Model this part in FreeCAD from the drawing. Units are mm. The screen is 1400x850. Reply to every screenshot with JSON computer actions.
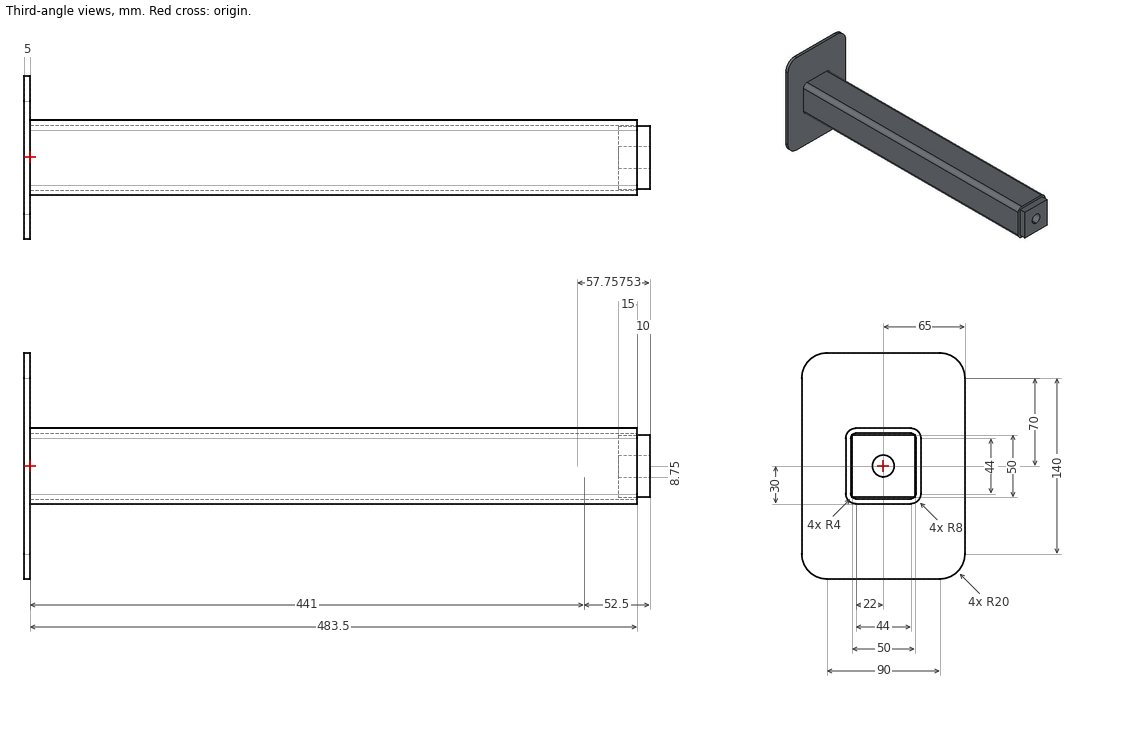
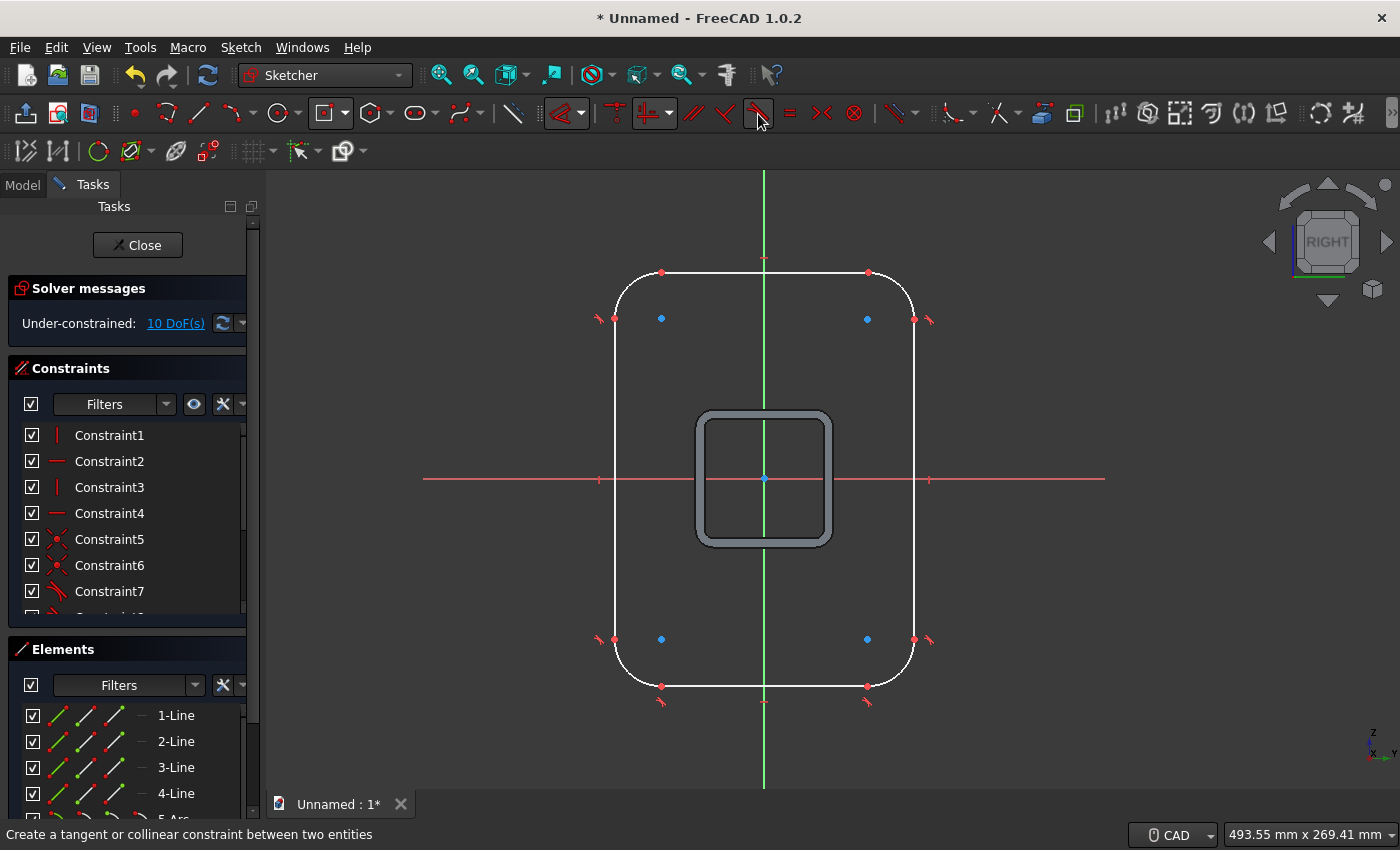
{"action": "left_click", "coordinate": [723, 273]}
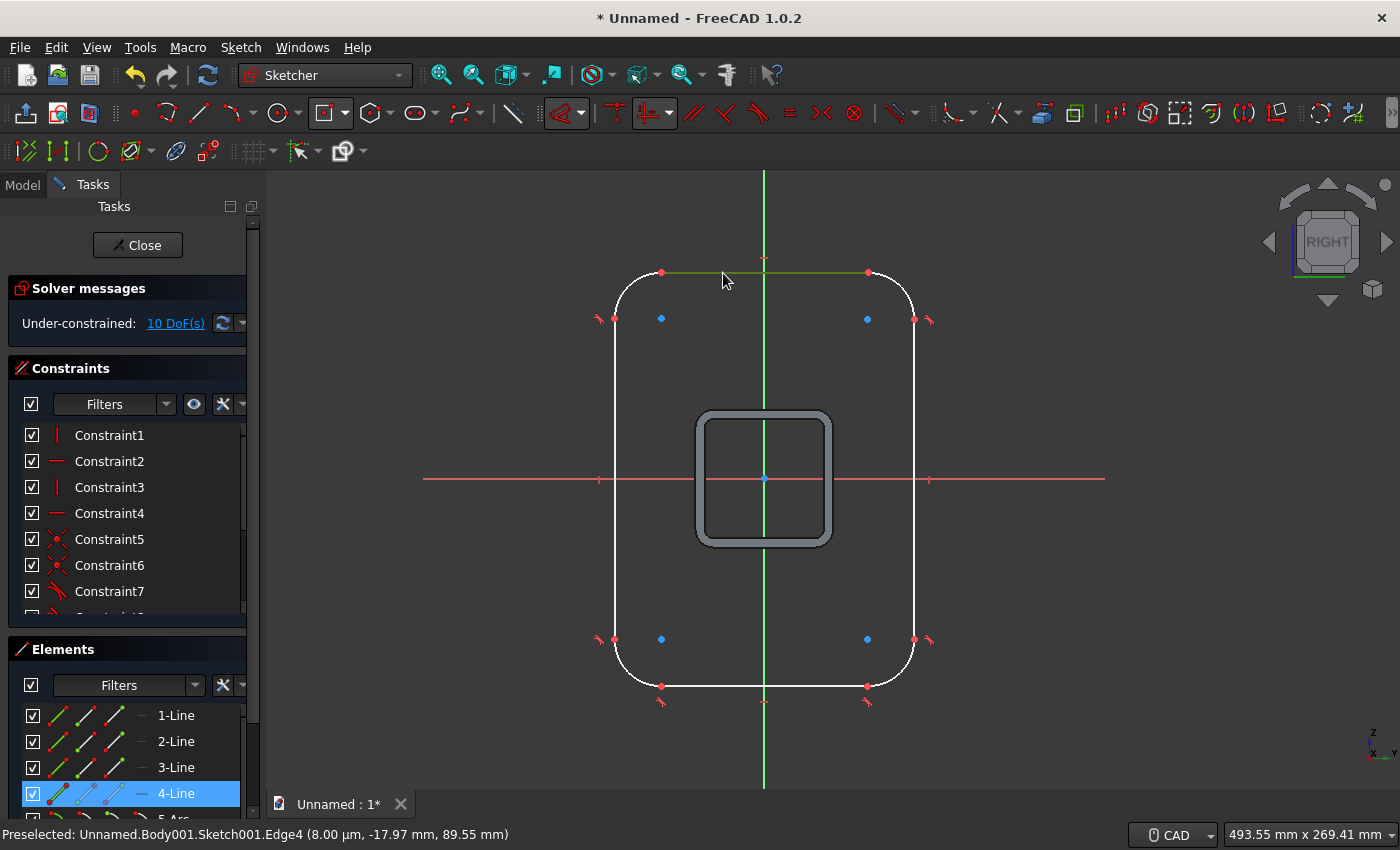
{"action": "left_click", "coordinate": [640, 278]}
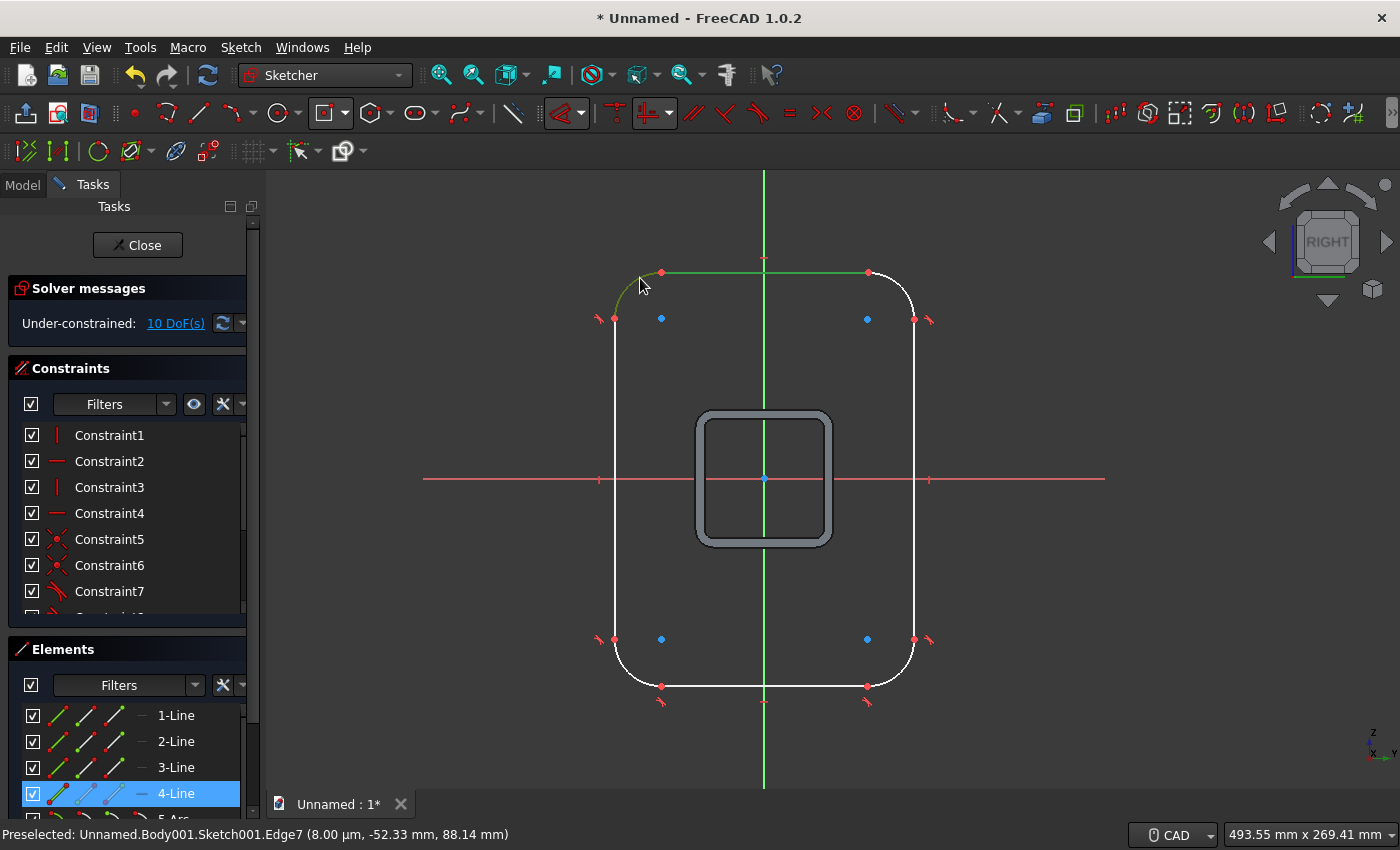
{"action": "left_click", "coordinate": [758, 114]}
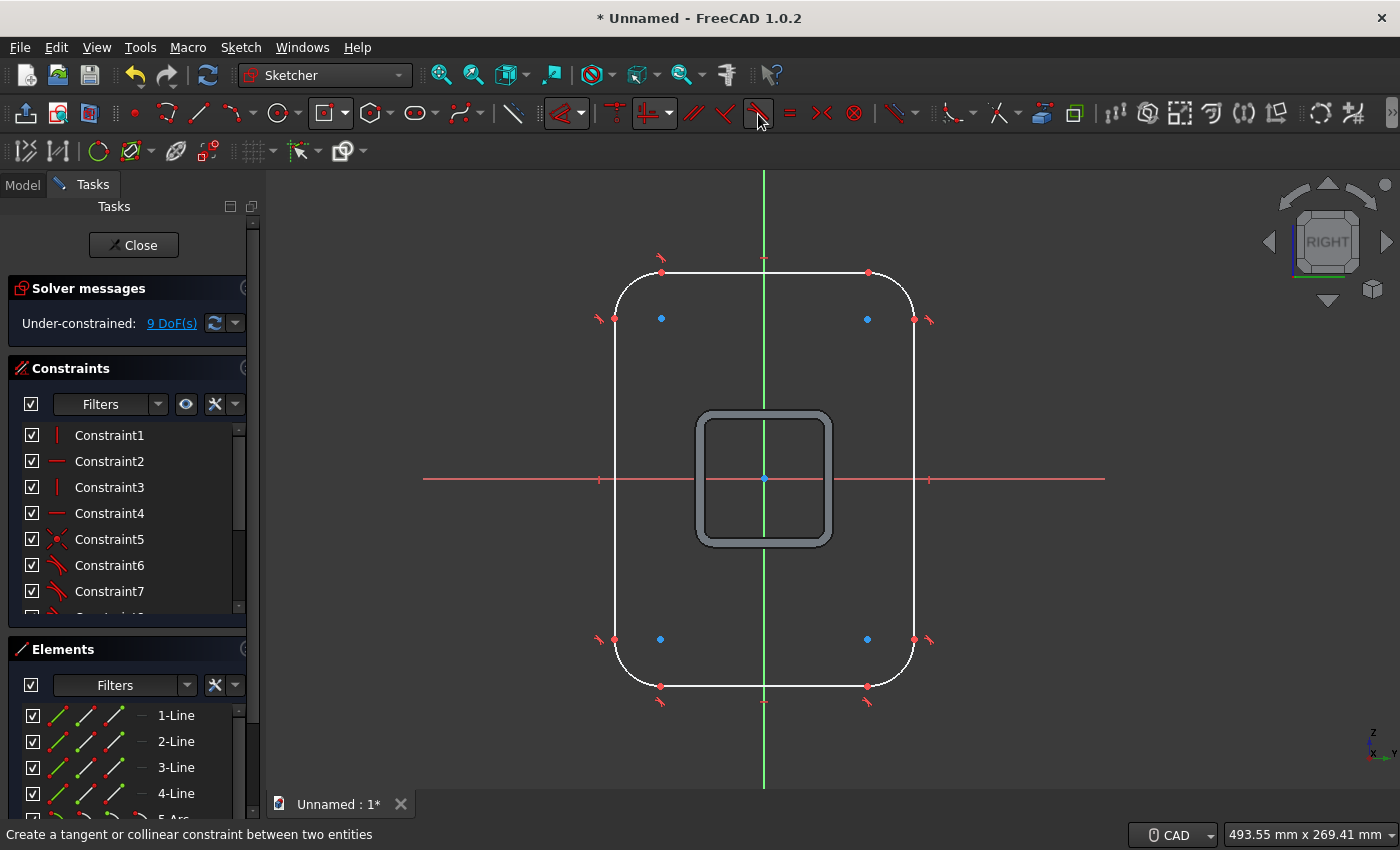
{"action": "left_click", "coordinate": [723, 273]}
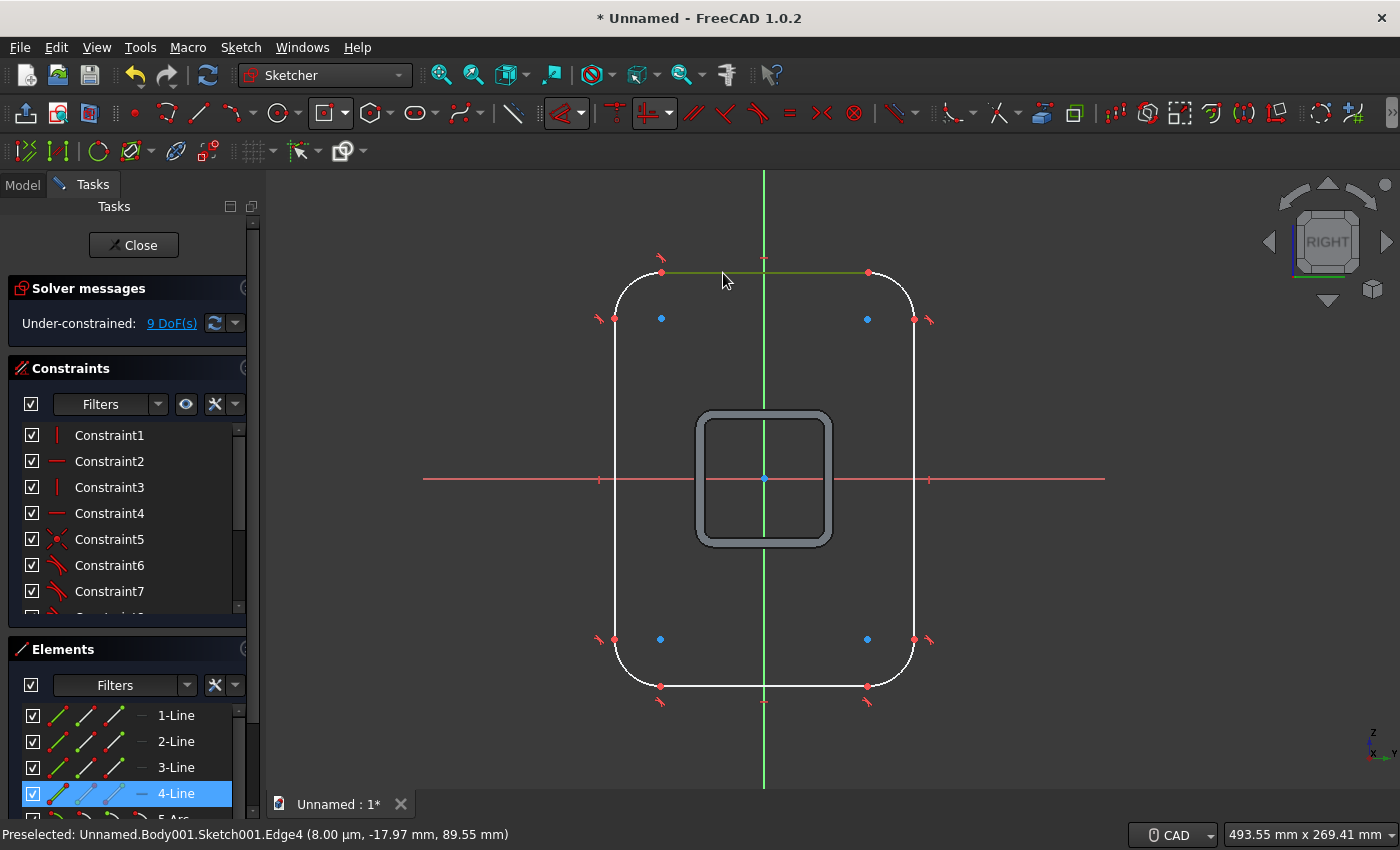
{"action": "left_click", "coordinate": [909, 298]}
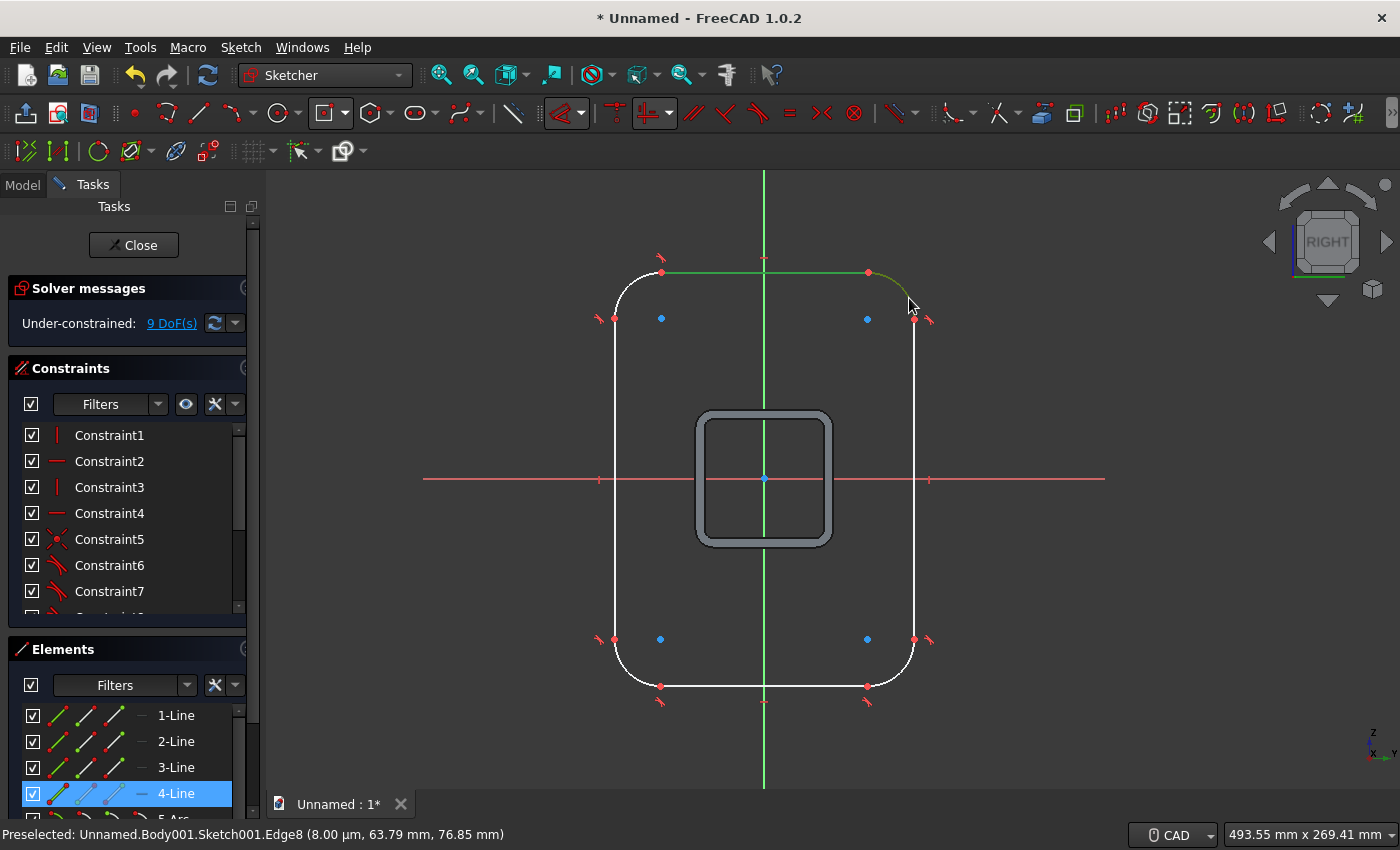
{"action": "left_click", "coordinate": [758, 114]}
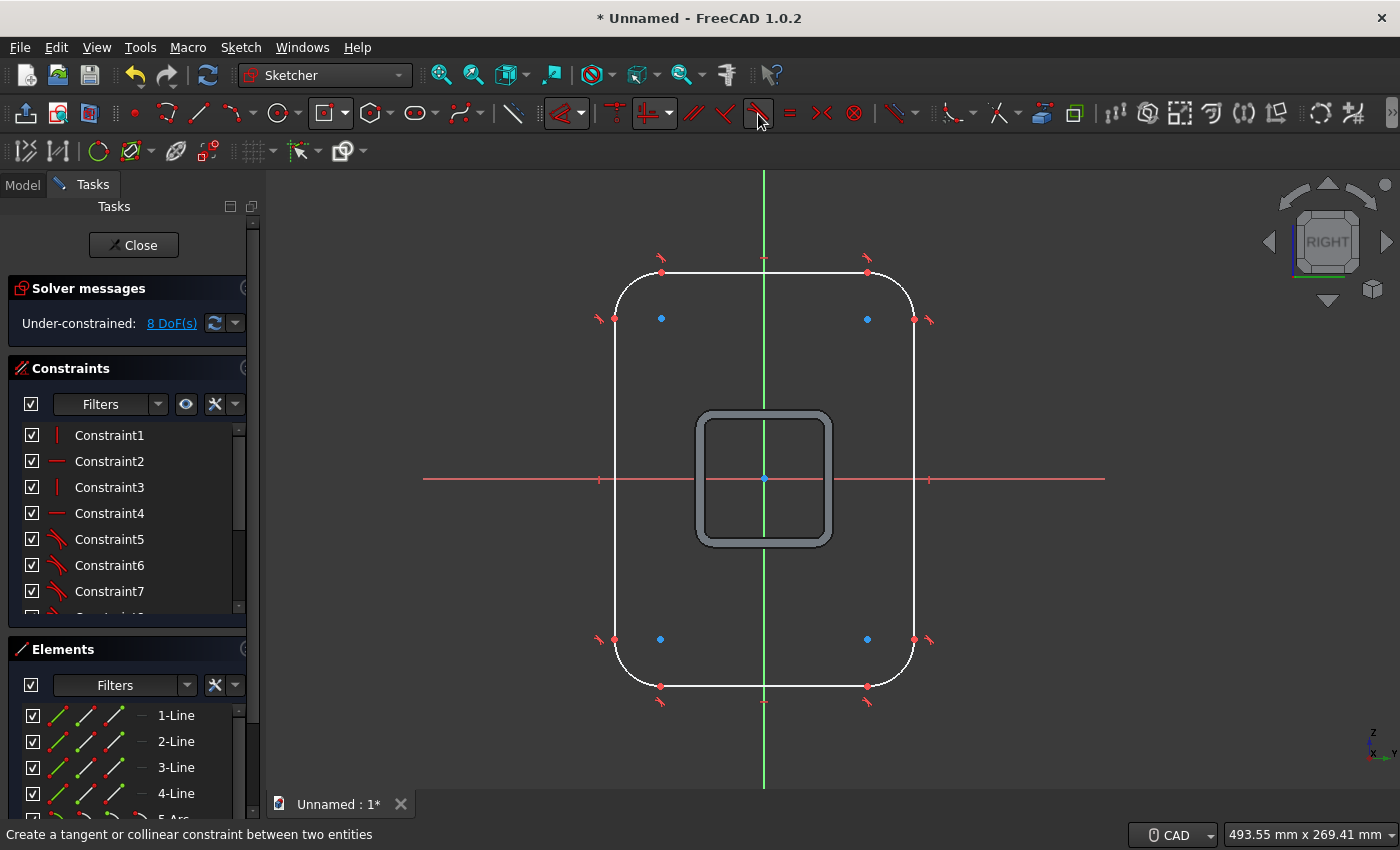
{"action": "left_click", "coordinate": [889, 681]}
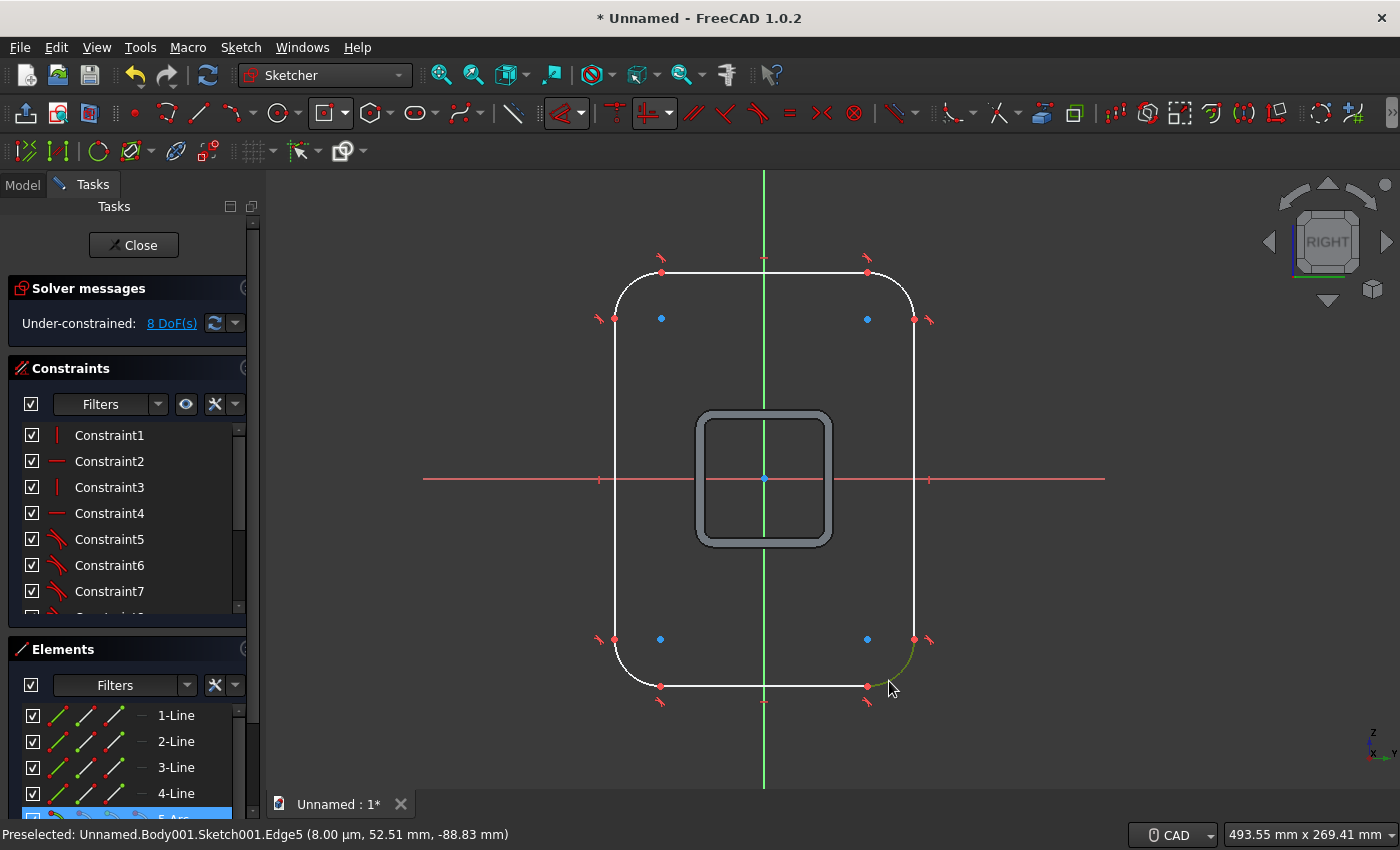
{"action": "left_click", "coordinate": [620, 661]}